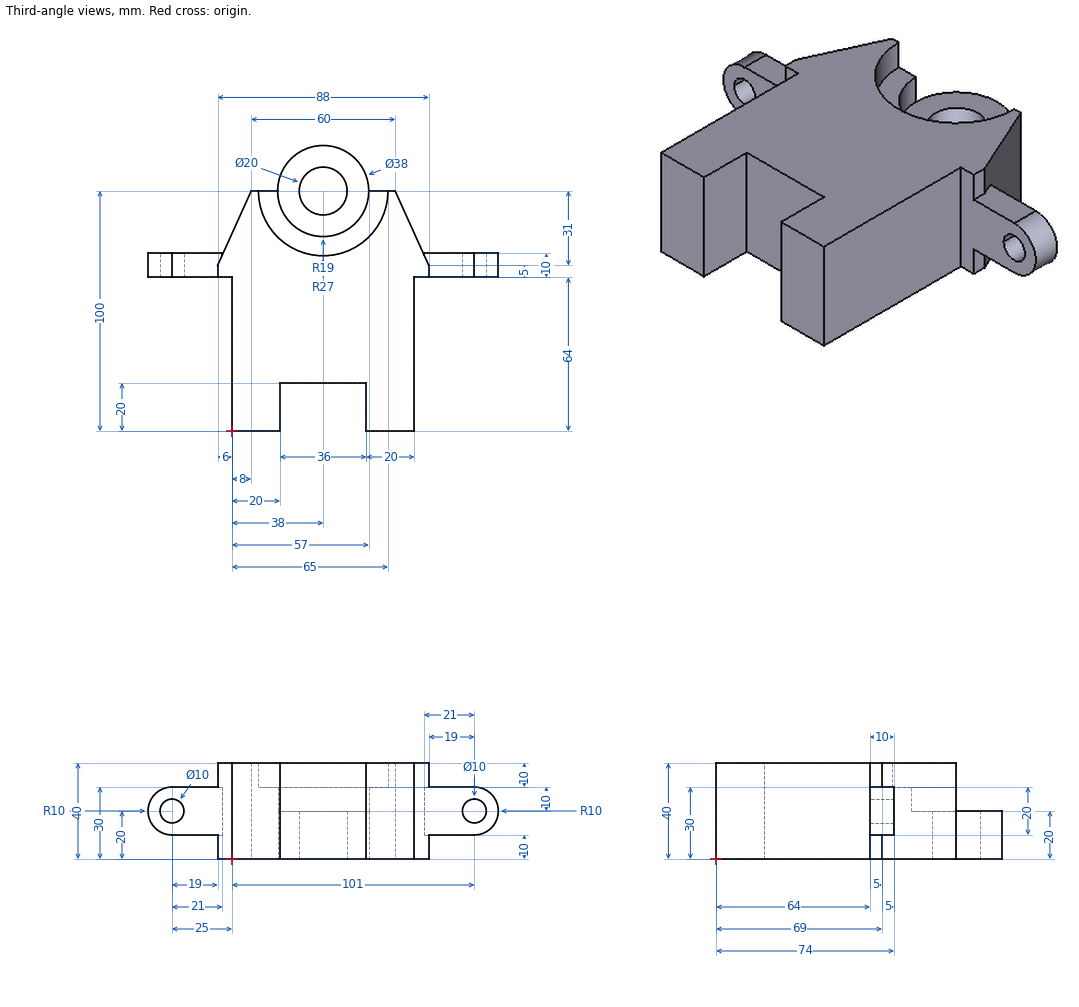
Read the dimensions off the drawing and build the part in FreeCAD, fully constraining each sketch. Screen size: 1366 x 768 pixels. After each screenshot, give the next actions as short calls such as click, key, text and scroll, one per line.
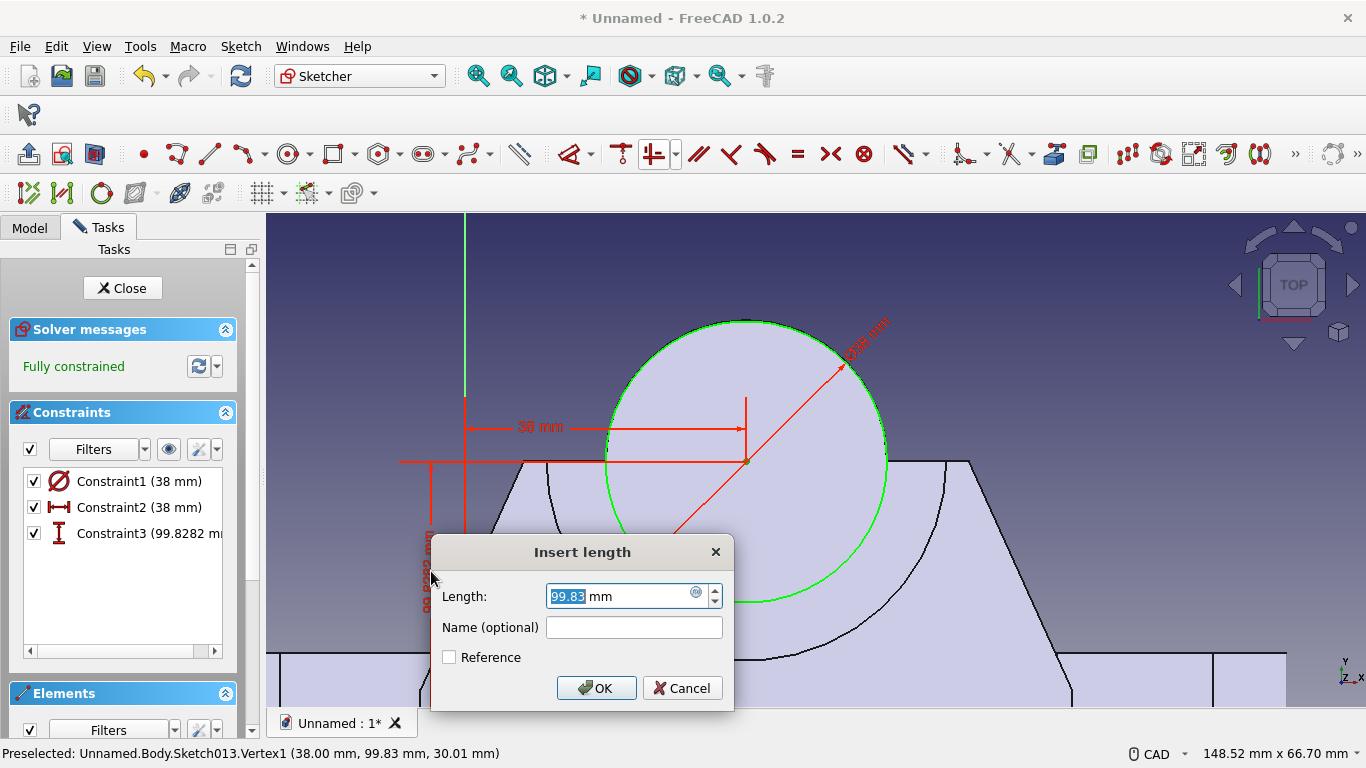
text(100)
key(Return)
key(Escape)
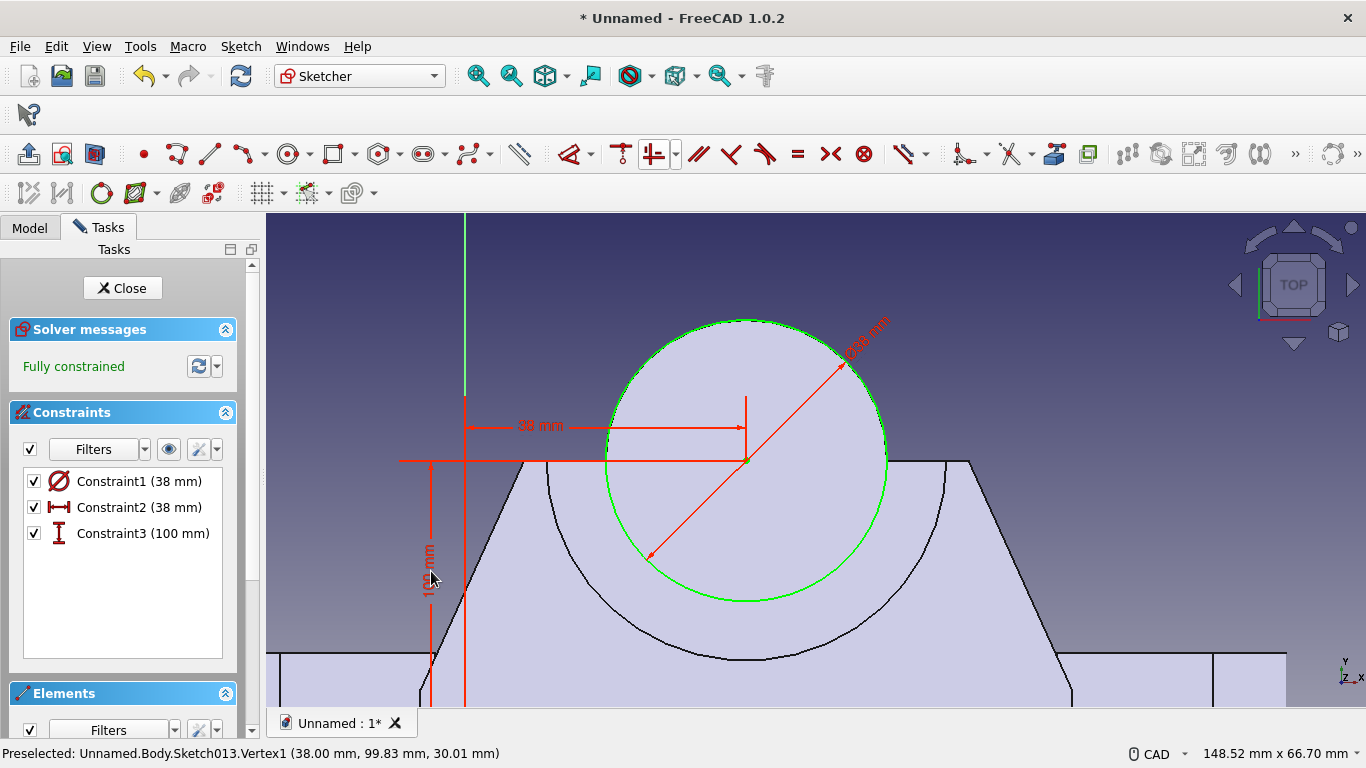
click(123, 288)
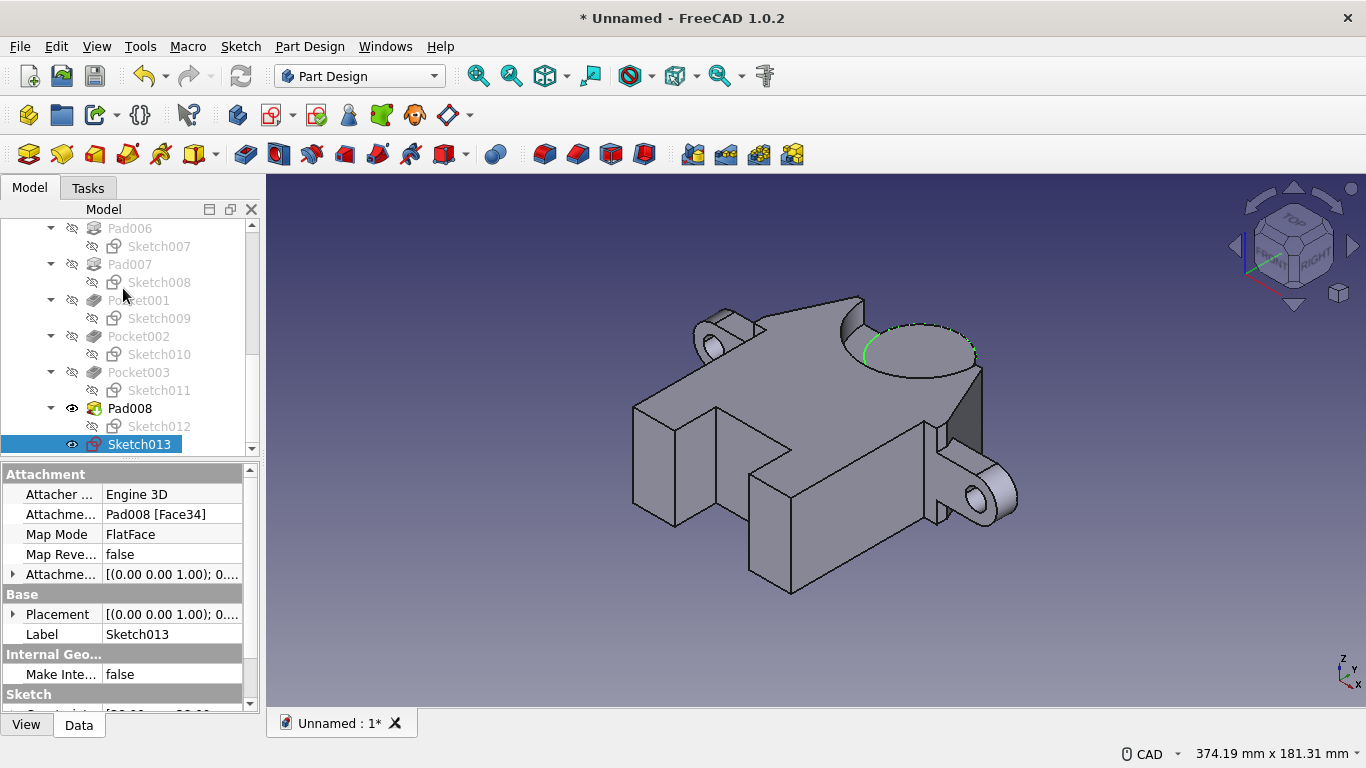
click(246, 154)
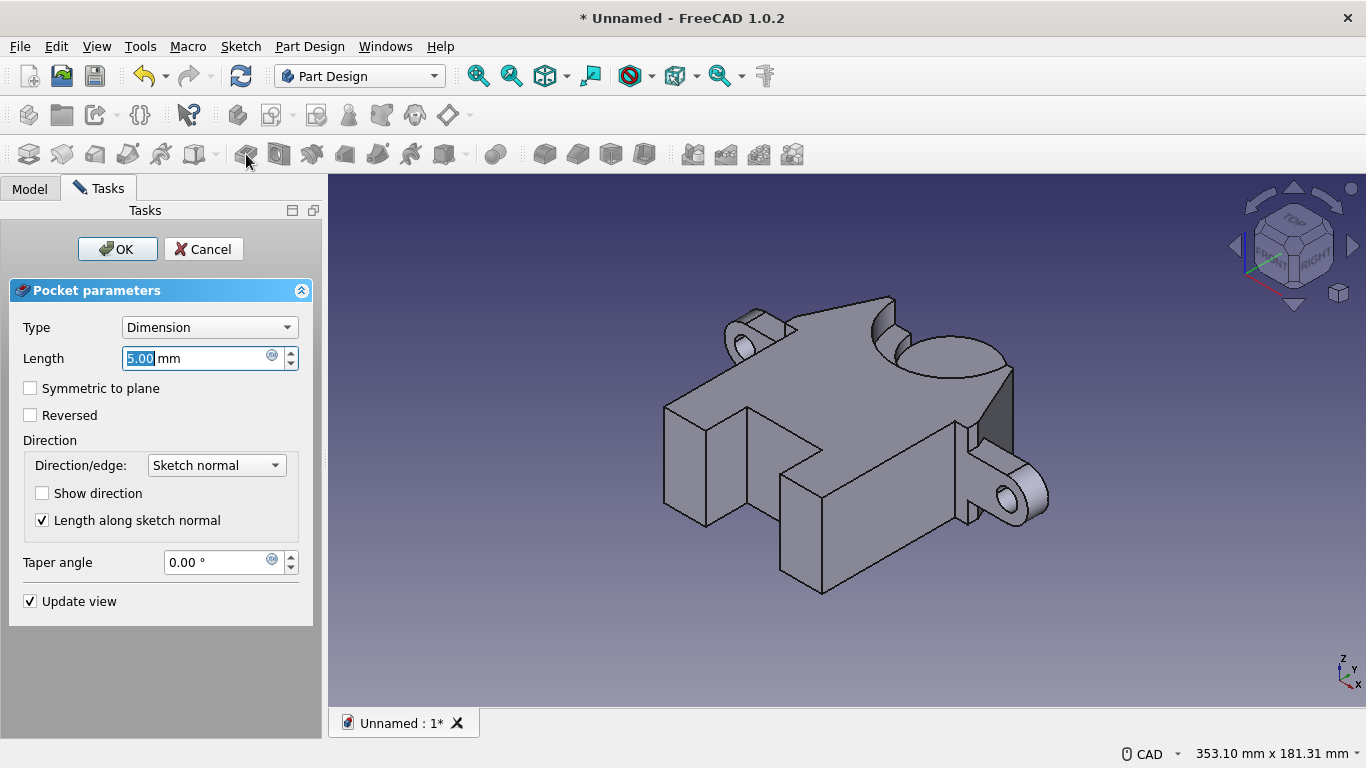
text(10)
key(Tab)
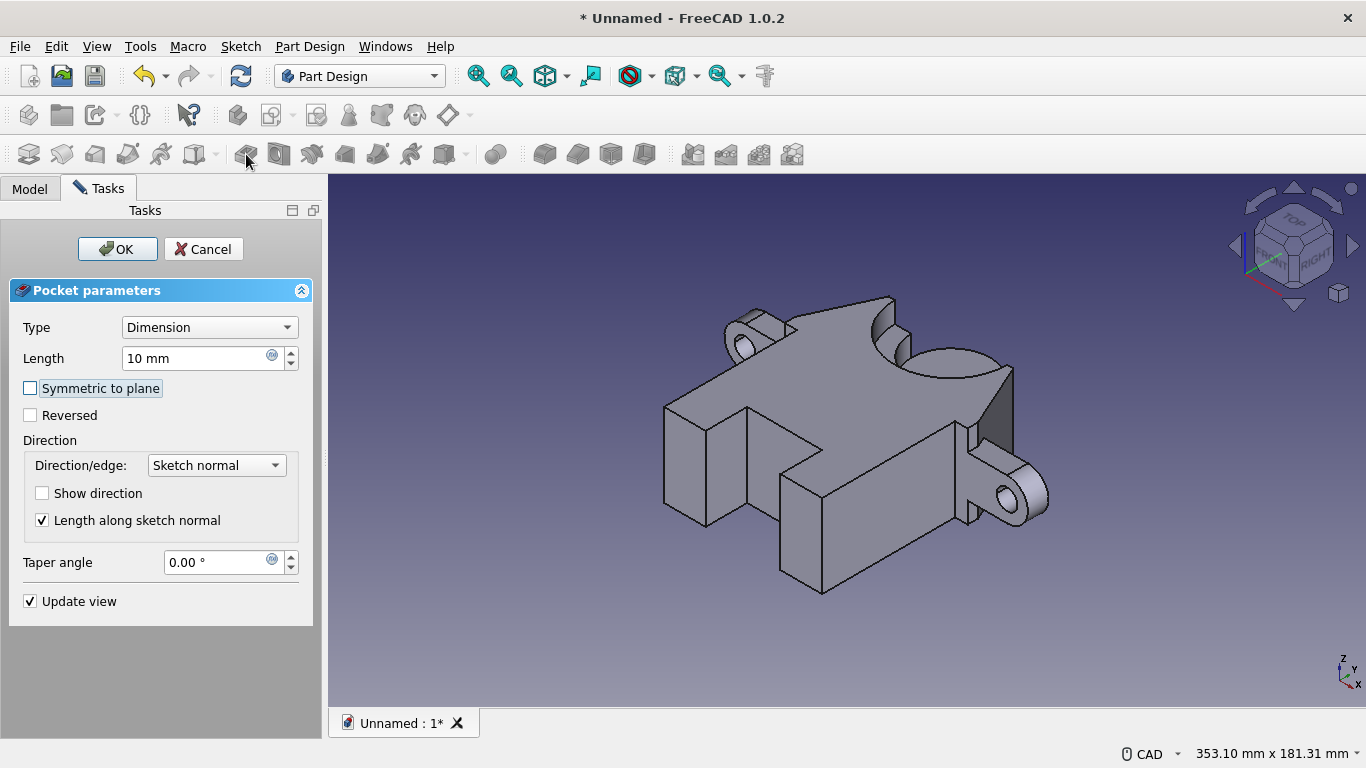
click(118, 249)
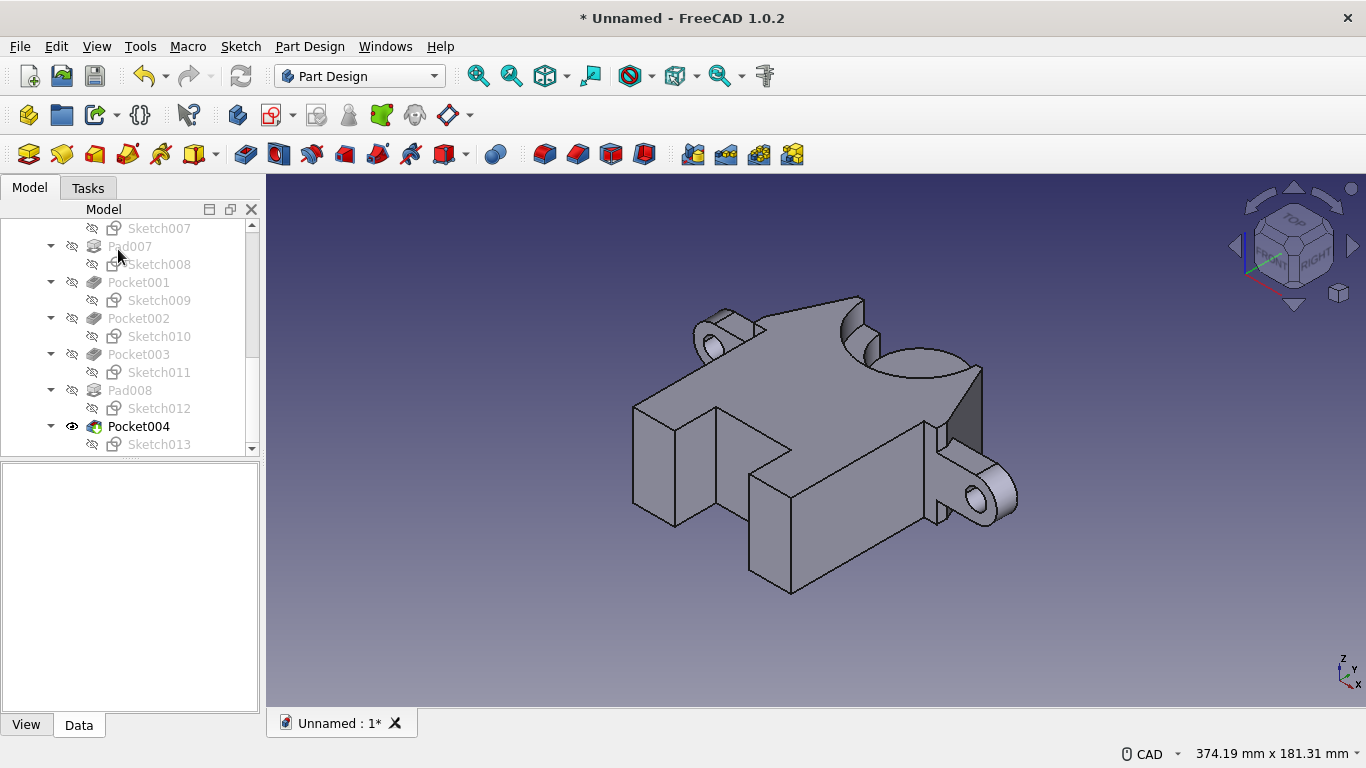
key(2)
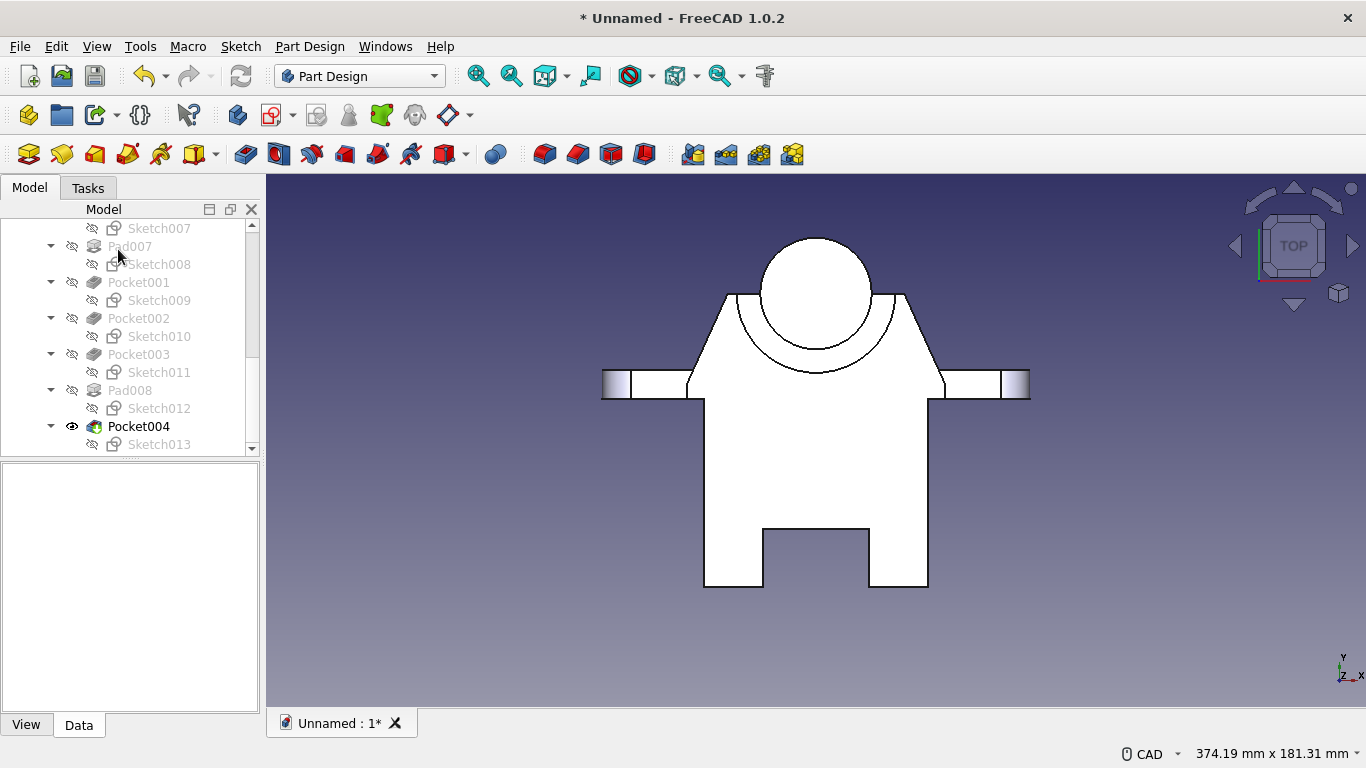
click(816, 293)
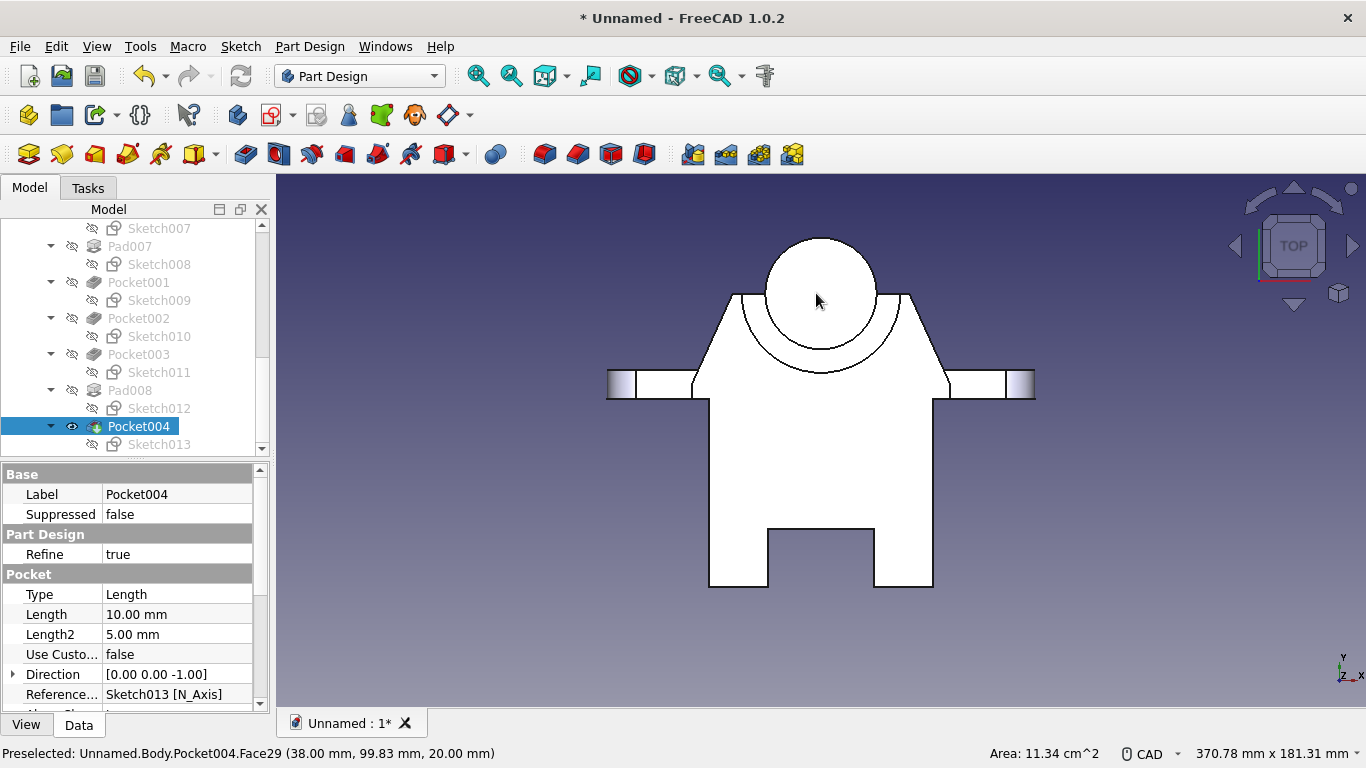
click(270, 116)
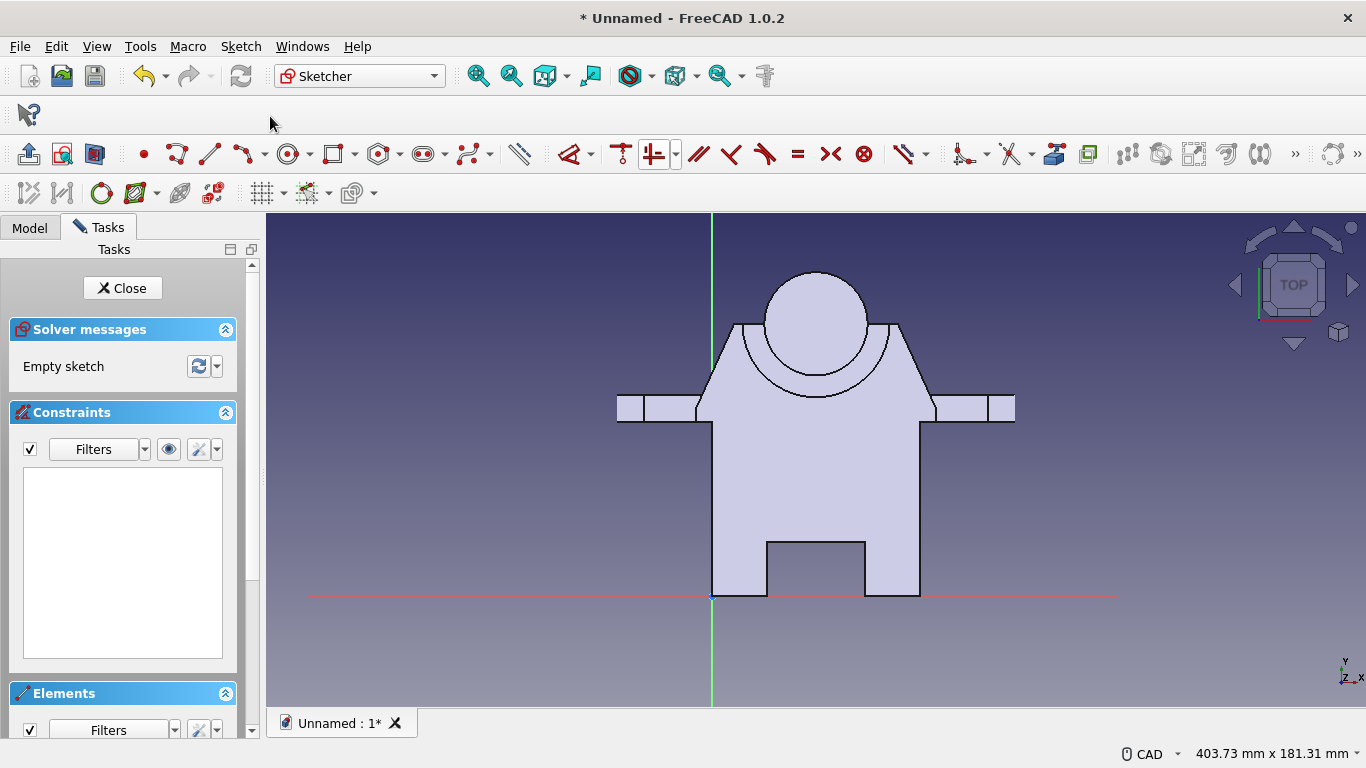
click(95, 154)